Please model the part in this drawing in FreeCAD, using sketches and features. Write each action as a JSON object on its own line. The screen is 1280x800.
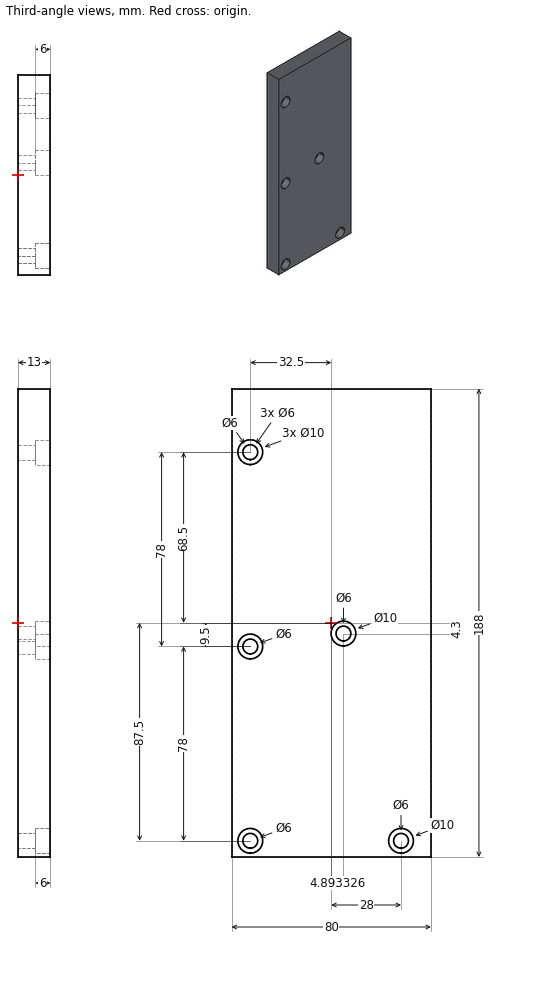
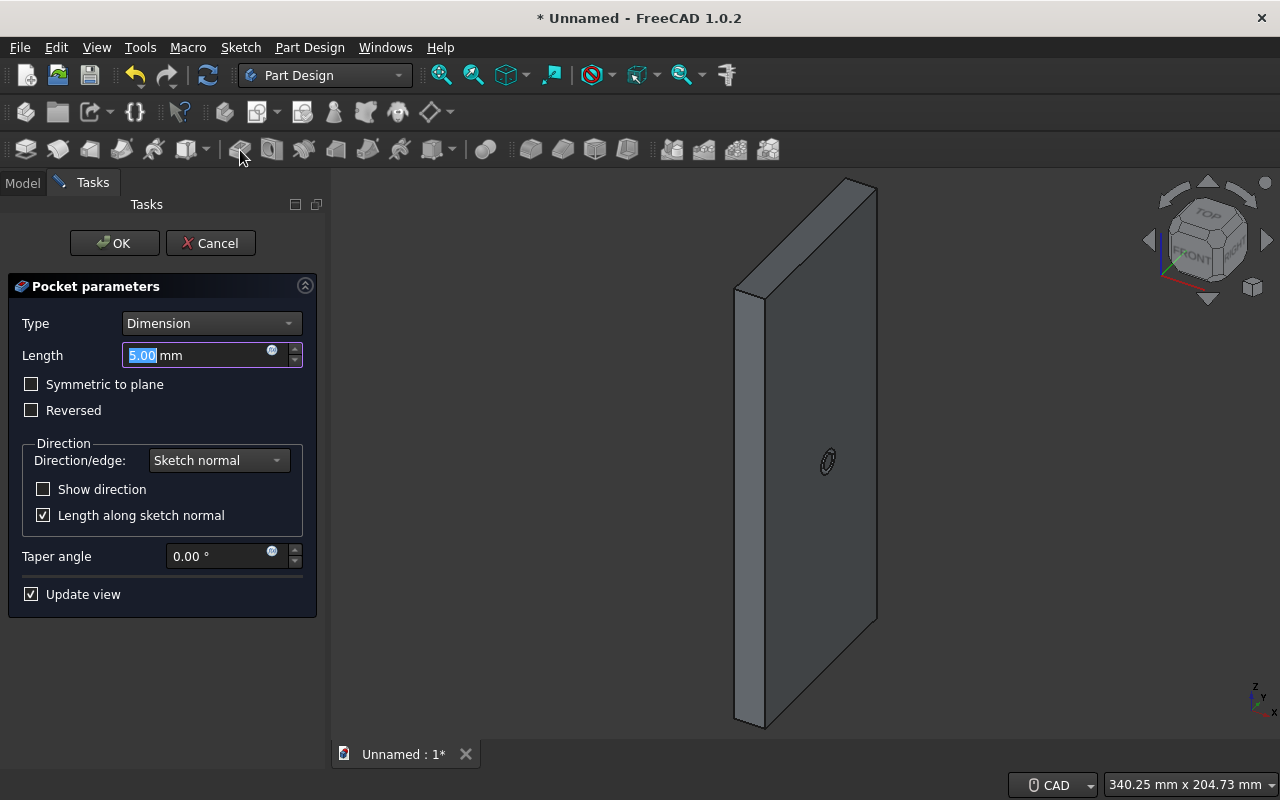
{"action": "type", "text": "6"}
{"action": "key", "text": "Tab"}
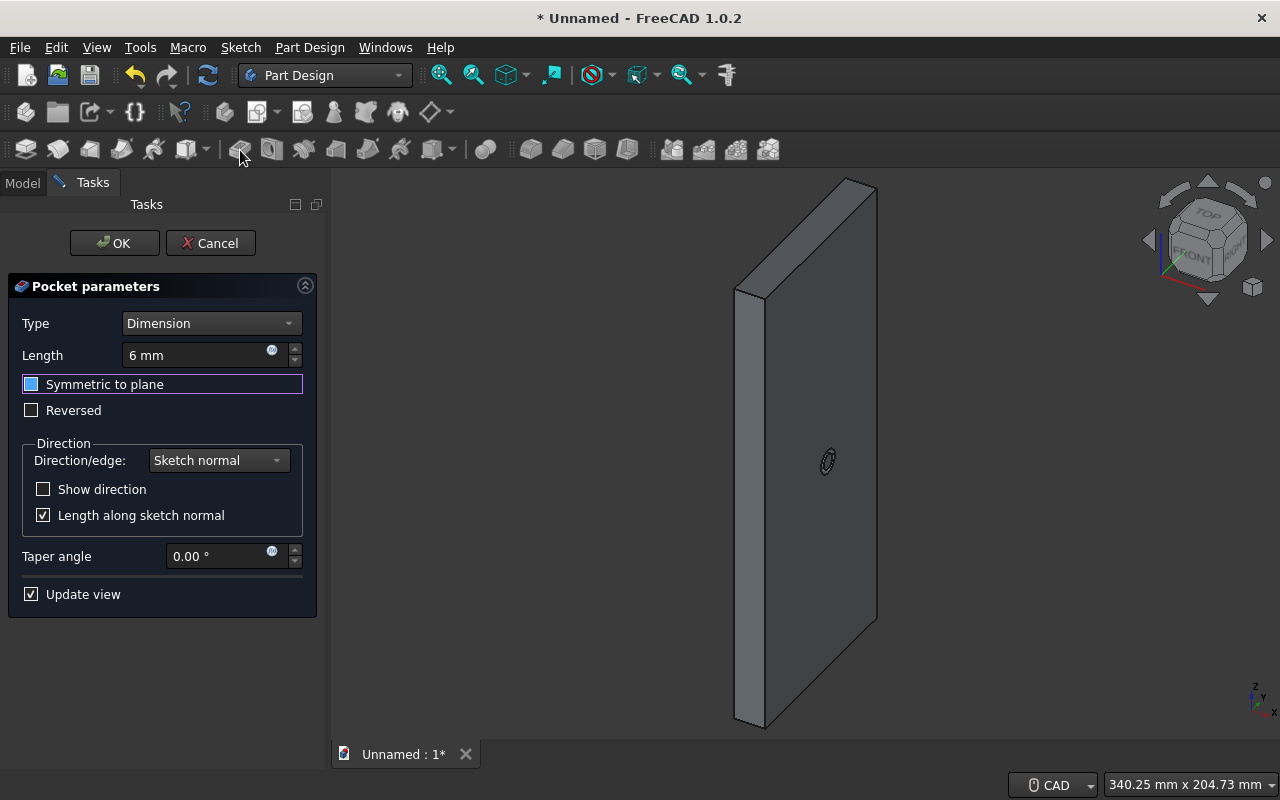
{"action": "left_click", "coordinate": [115, 243]}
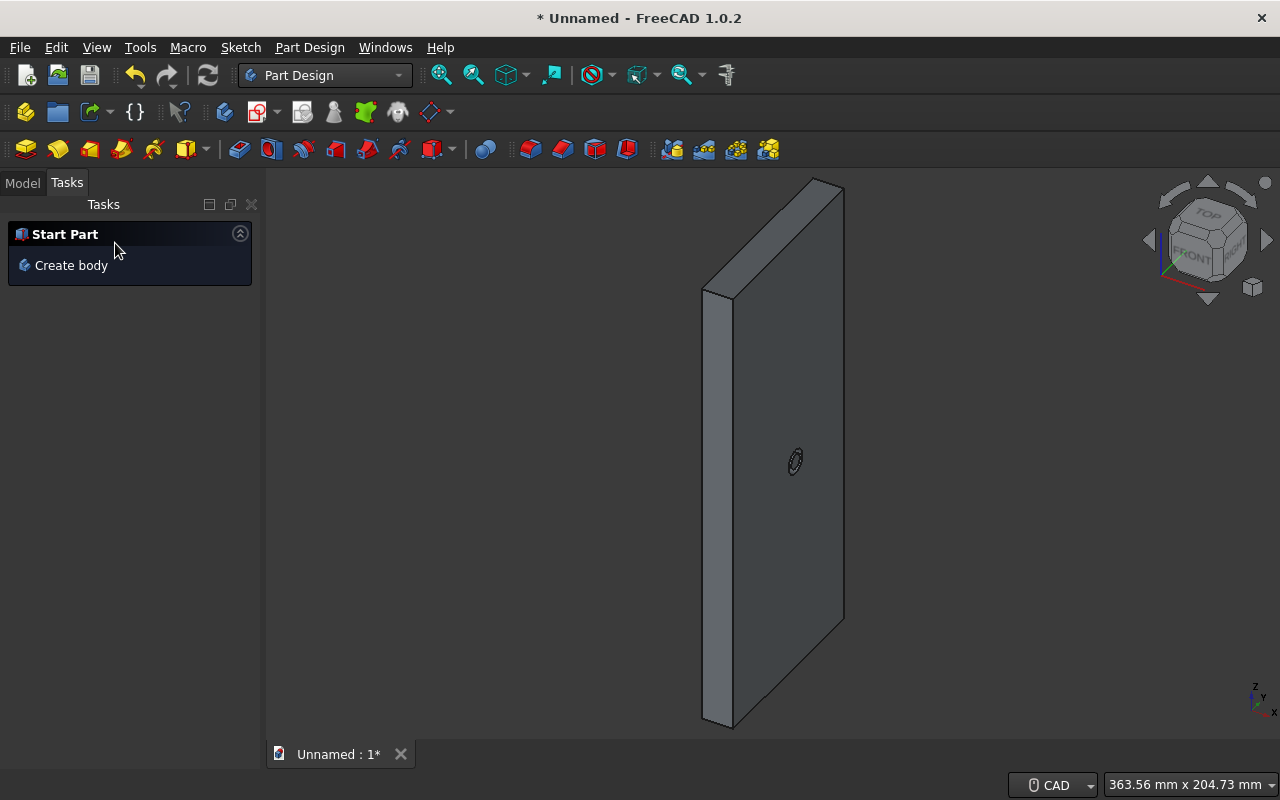
{"action": "left_click", "coordinate": [789, 335]}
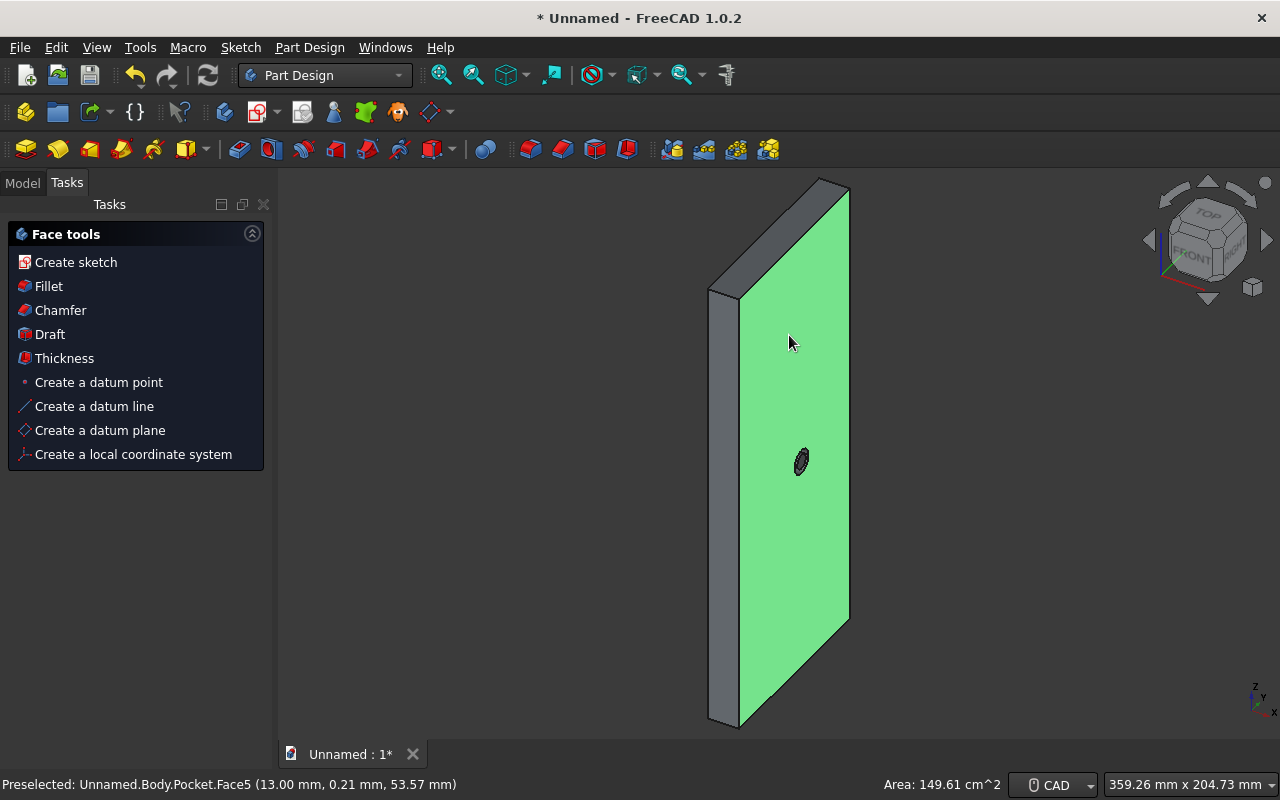
{"action": "left_click", "coordinate": [258, 112]}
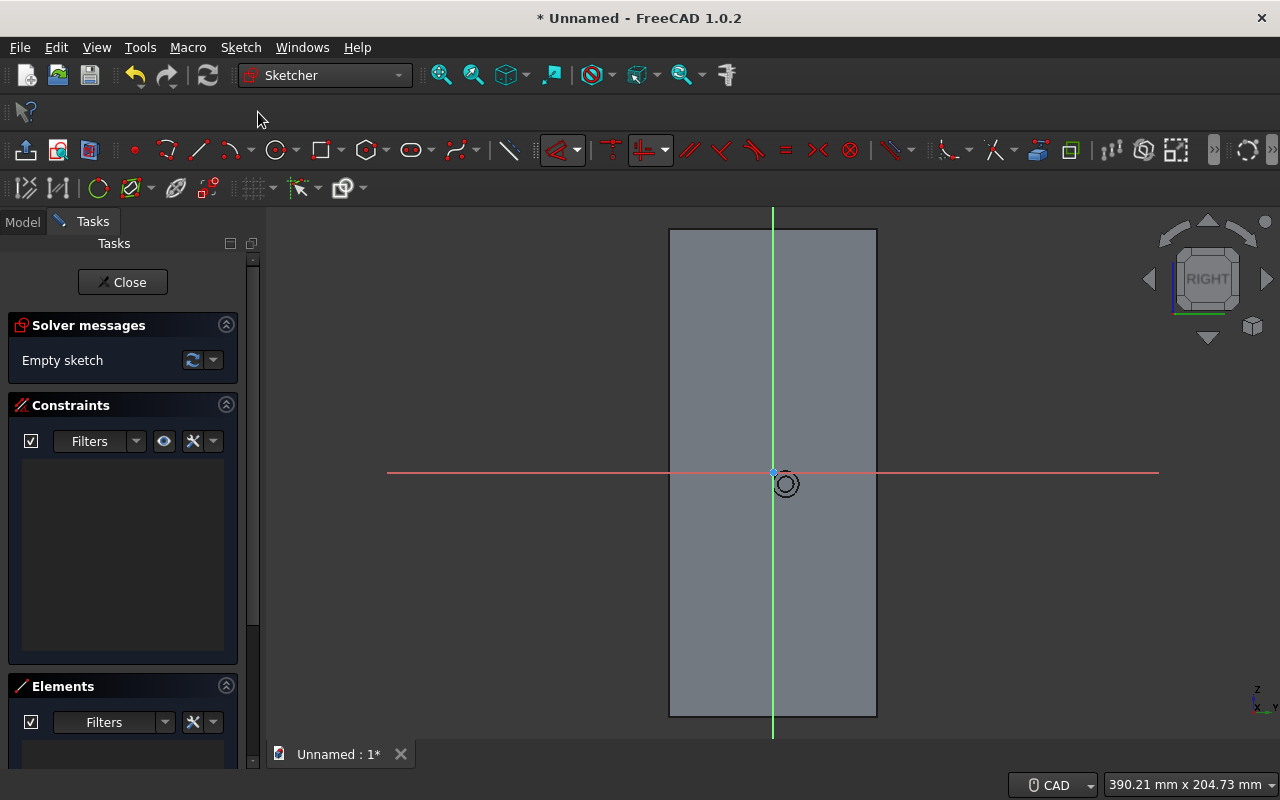
{"action": "scroll", "coordinate": [788, 483], "scroll_direction": "up", "scroll_amount": 14}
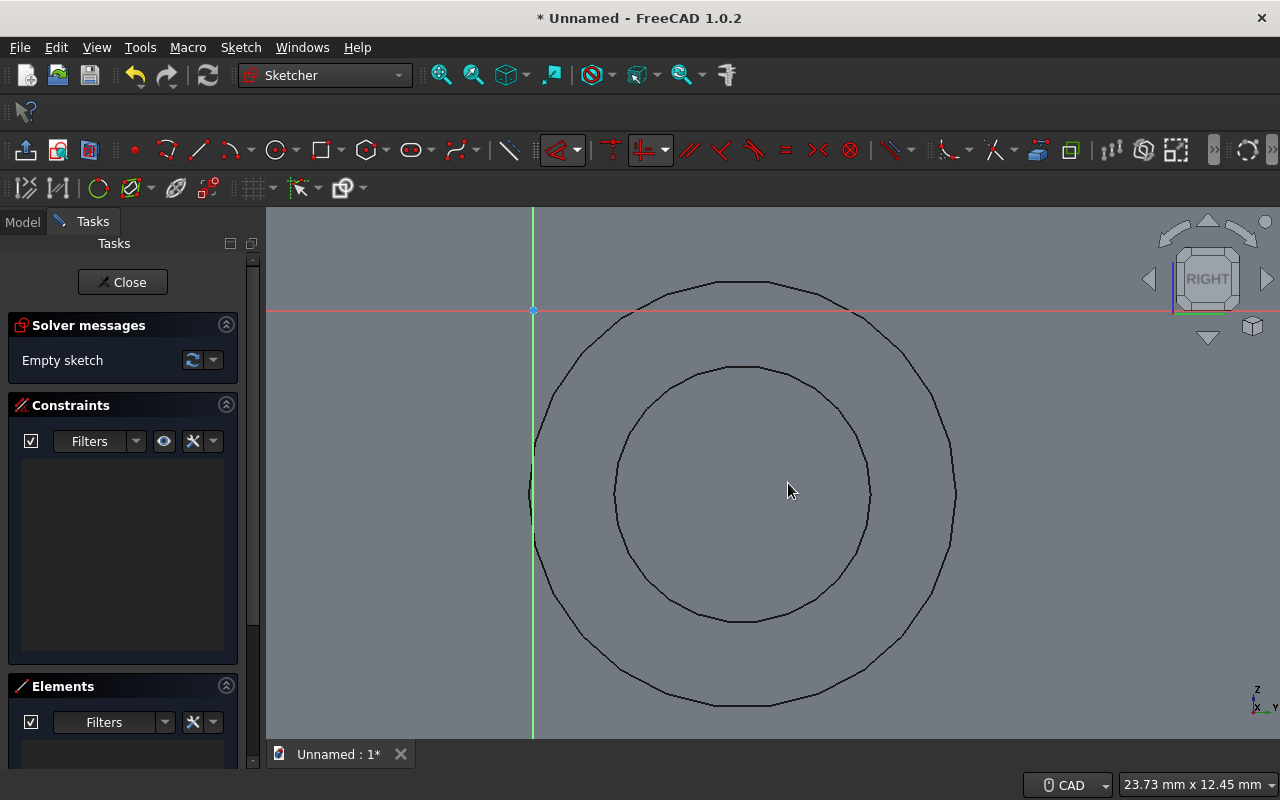
{"action": "left_click", "coordinate": [276, 150]}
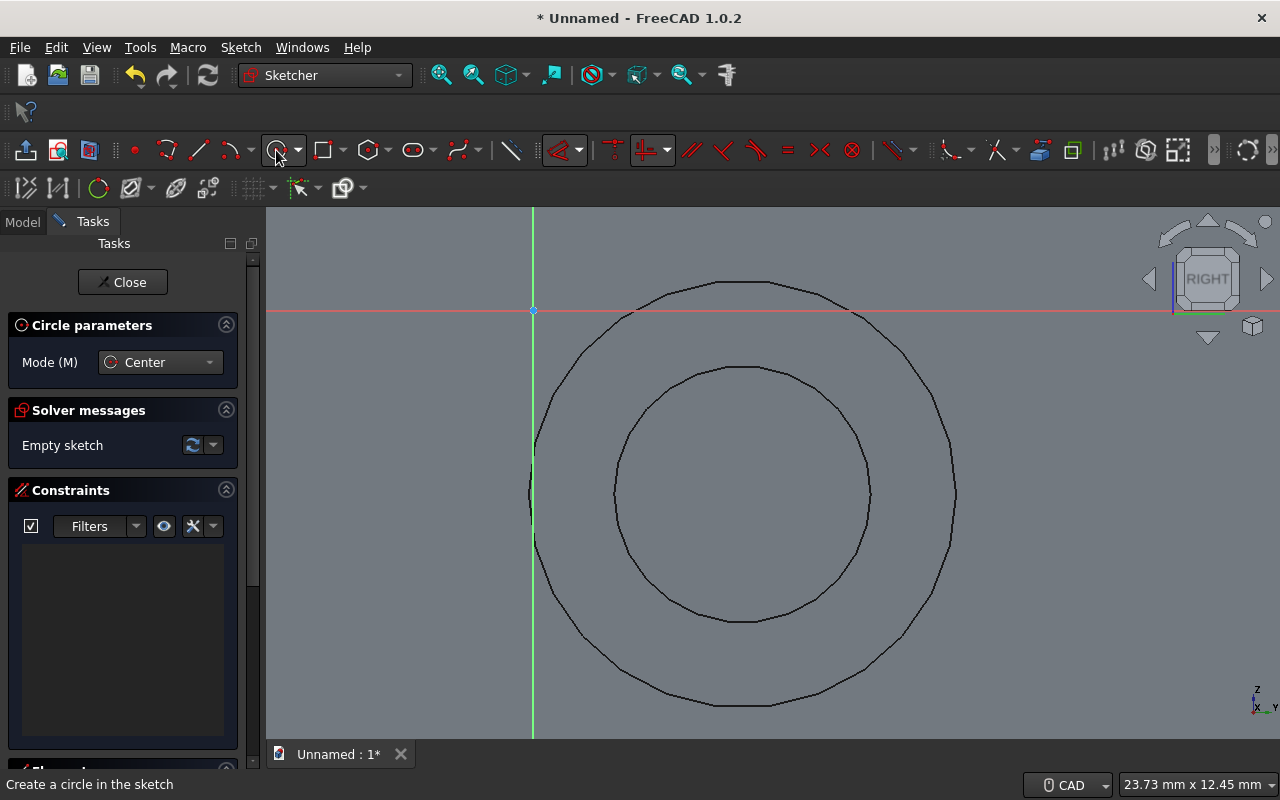
{"action": "left_click", "coordinate": [742, 494]}
{"action": "left_click", "coordinate": [833, 404]}
{"action": "key", "text": "Escape"}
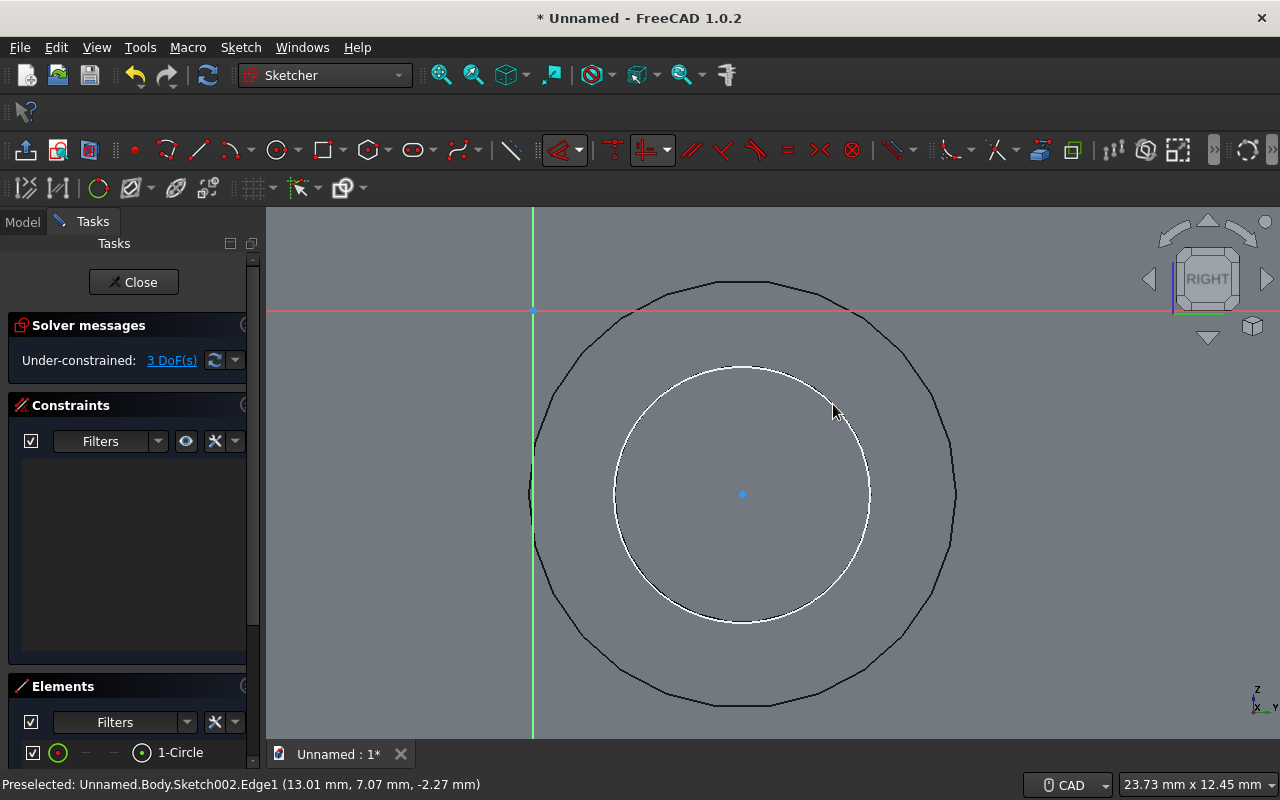
{"action": "left_click", "coordinate": [832, 404]}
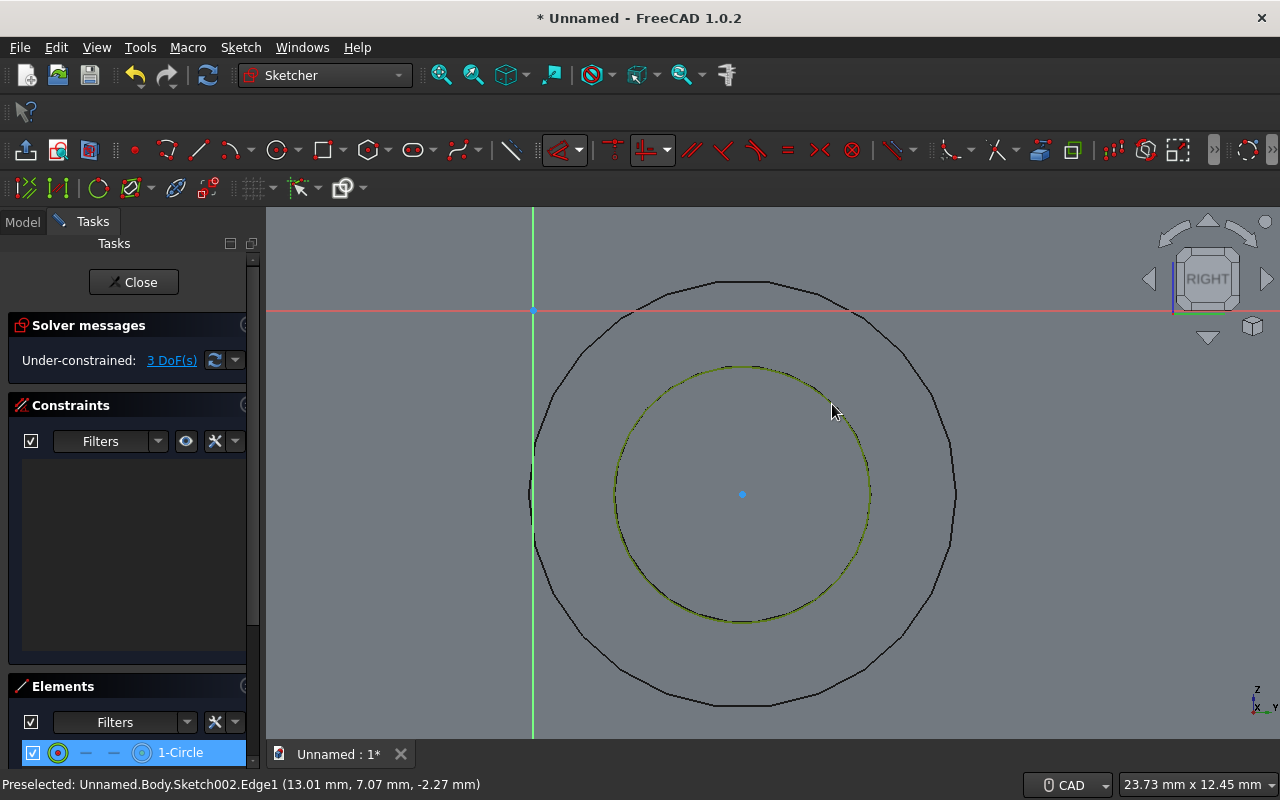
{"action": "left_click", "coordinate": [582, 150]}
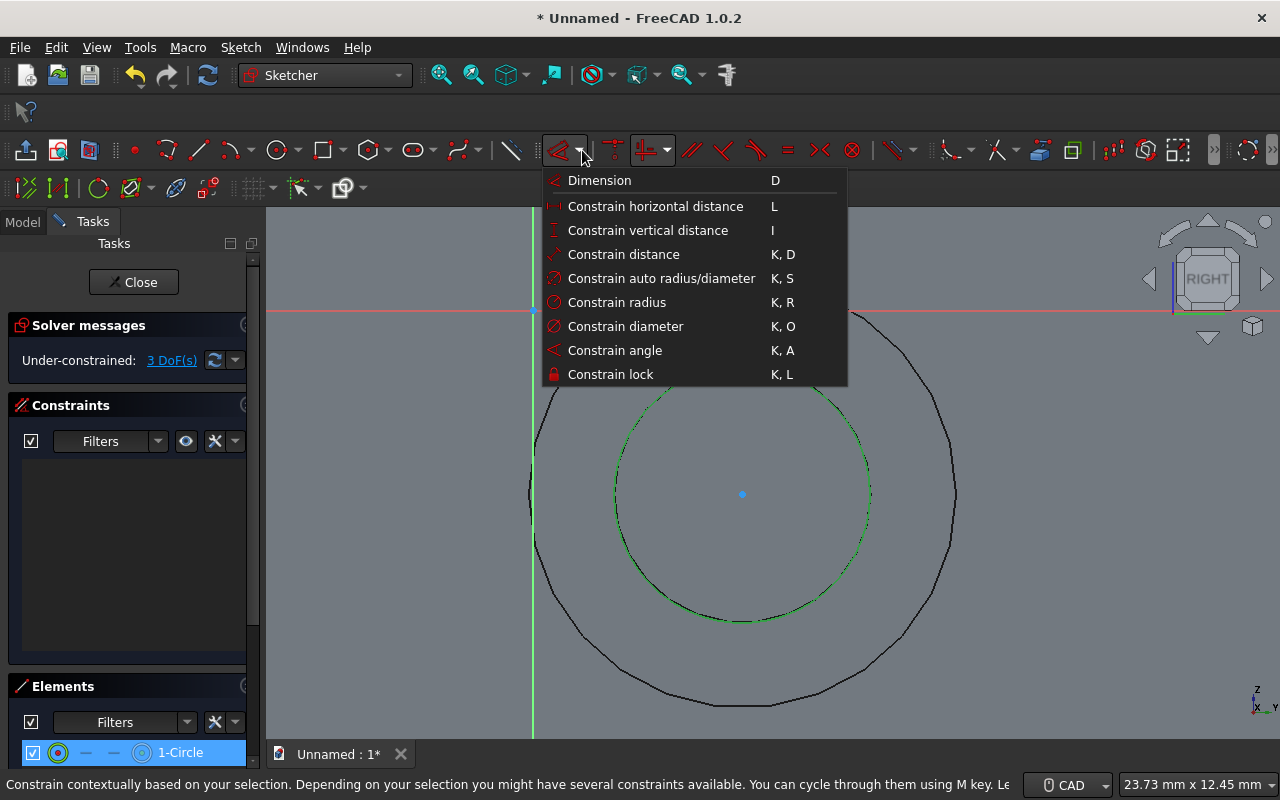
{"action": "left_click", "coordinate": [695, 326]}